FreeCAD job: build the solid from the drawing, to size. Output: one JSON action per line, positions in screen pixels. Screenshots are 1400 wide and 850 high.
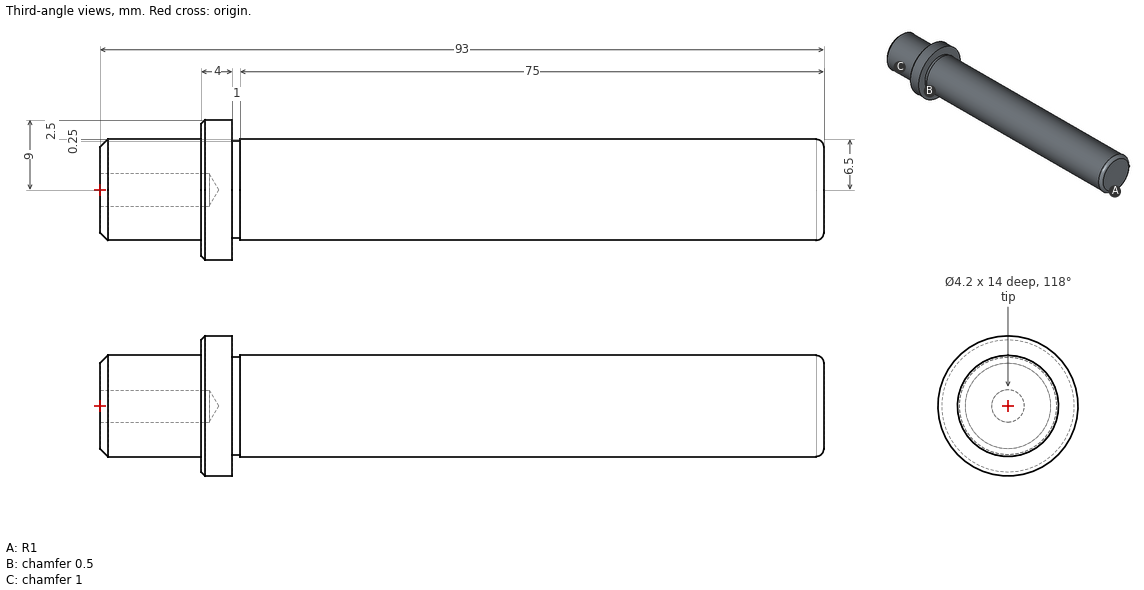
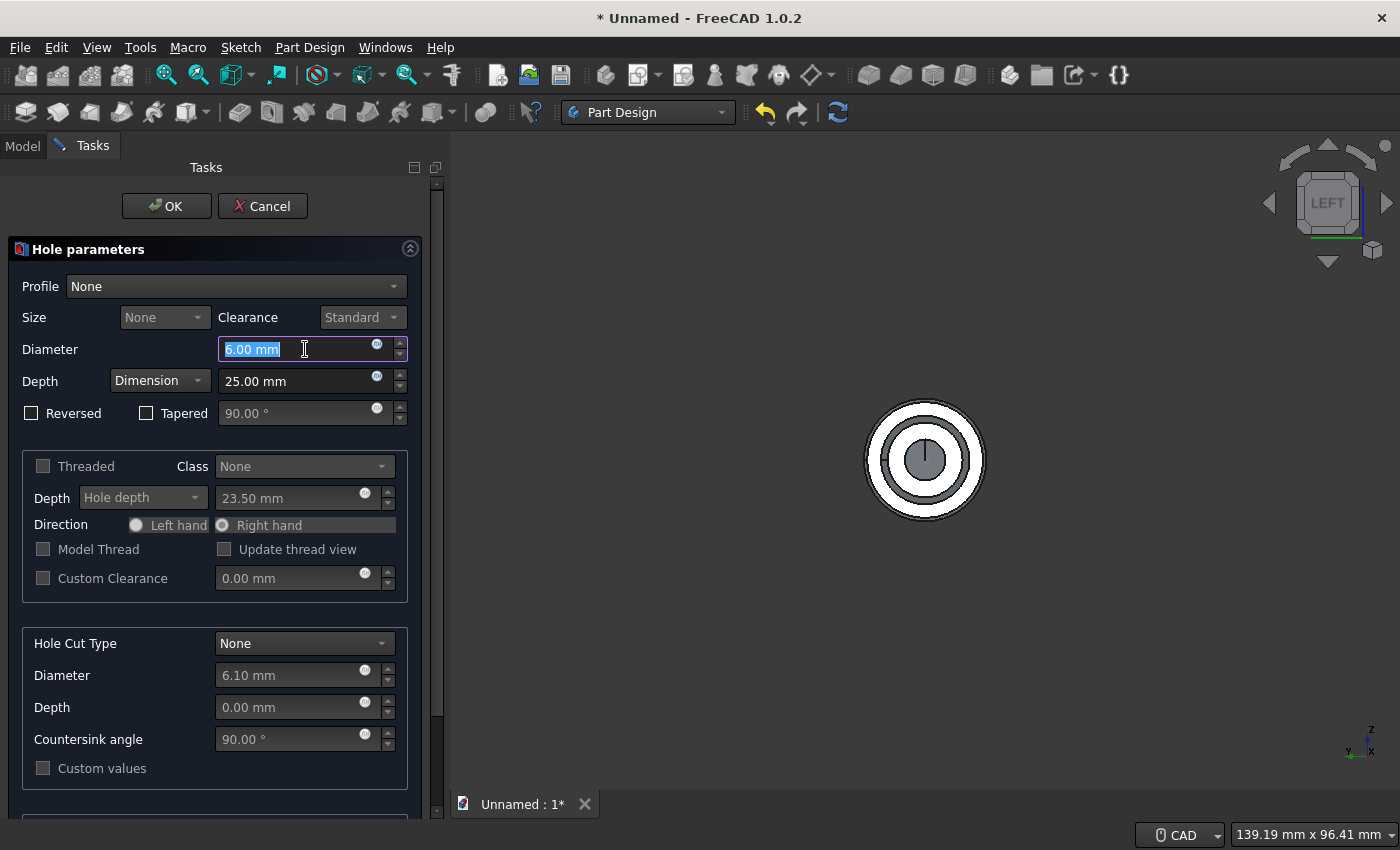
{"action": "type", "text": "4.2"}
{"action": "key", "text": "Tab"}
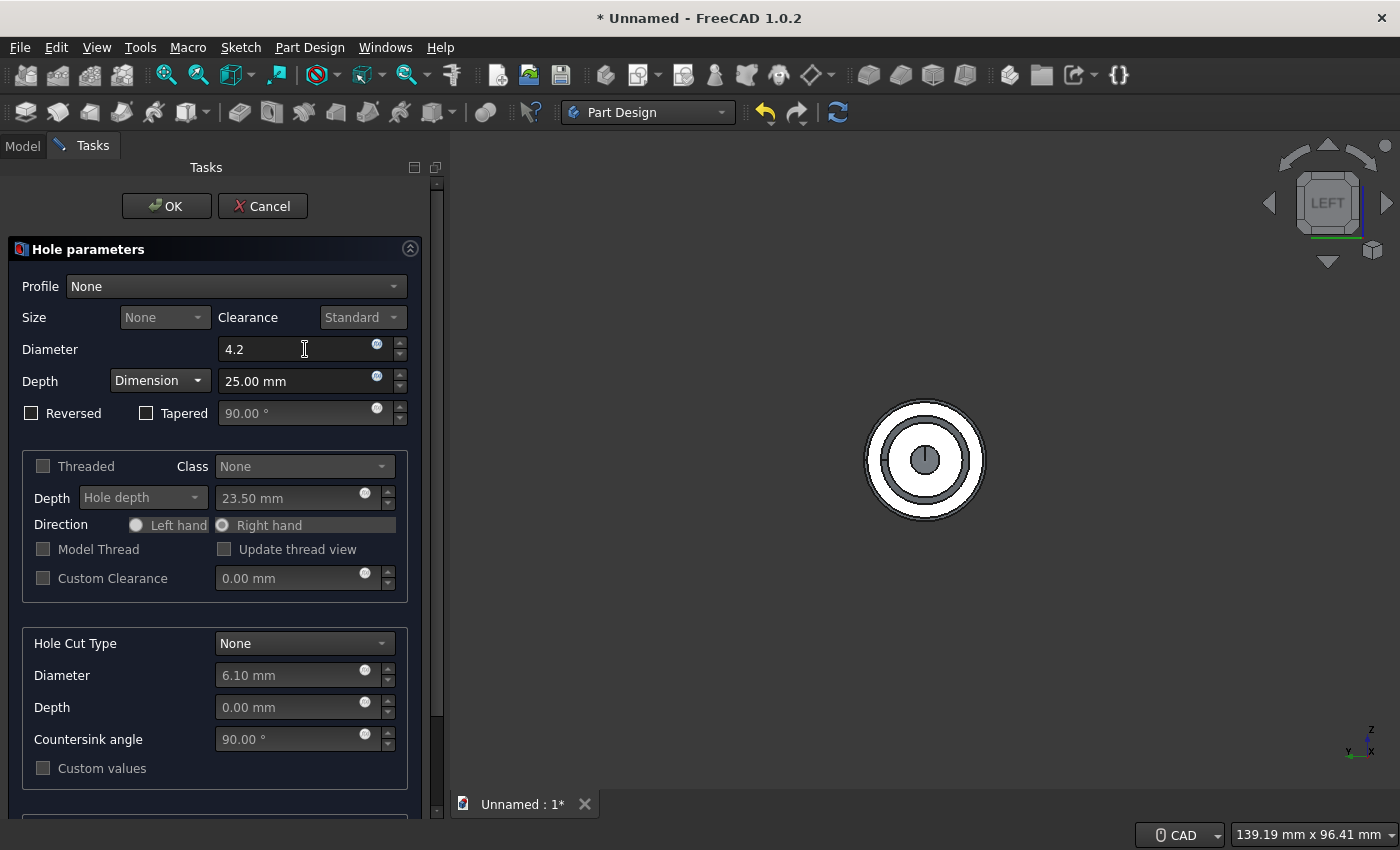
{"action": "triple_click", "coordinate": [305, 381]}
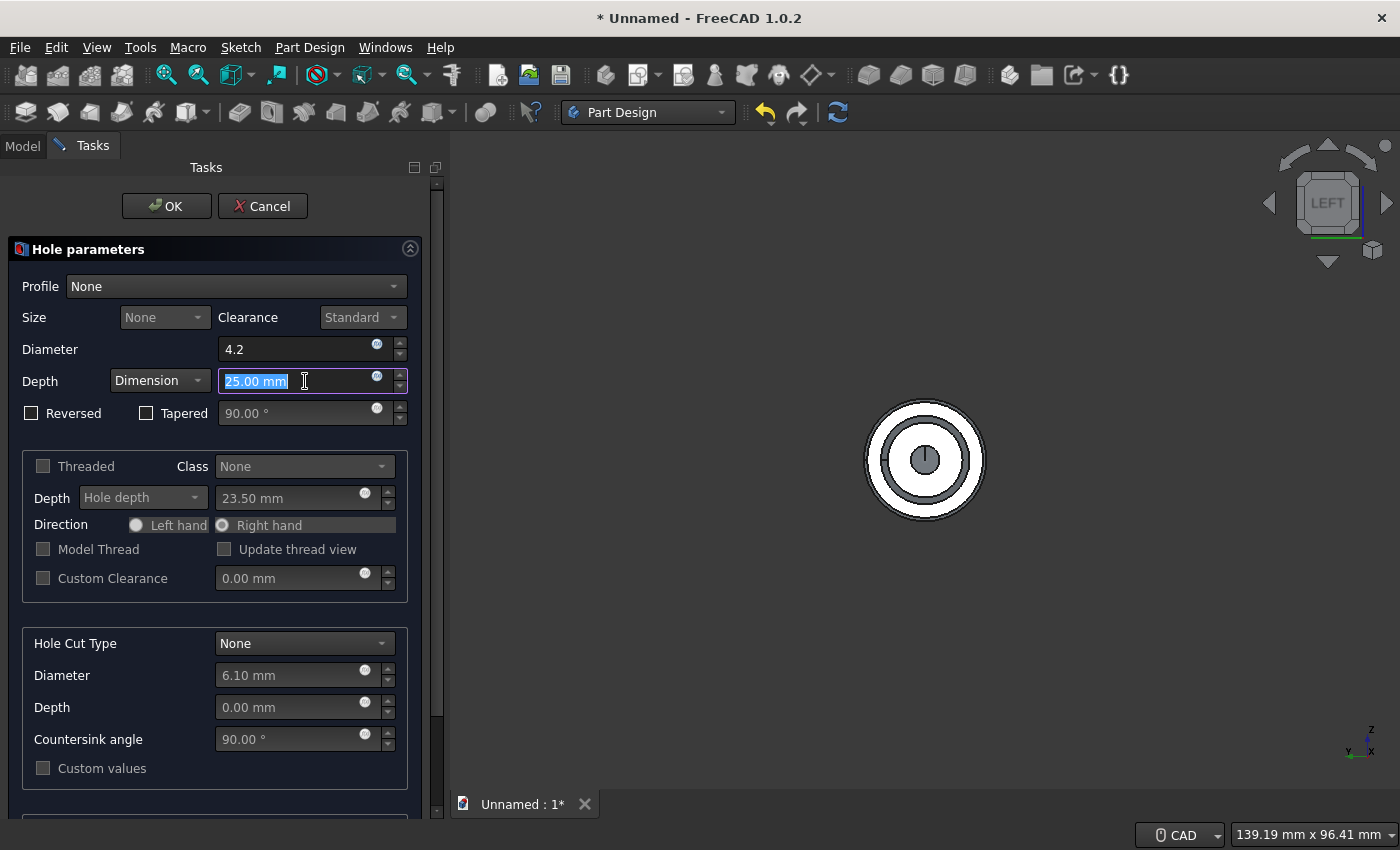
{"action": "type", "text": "14"}
{"action": "key", "text": "Tab"}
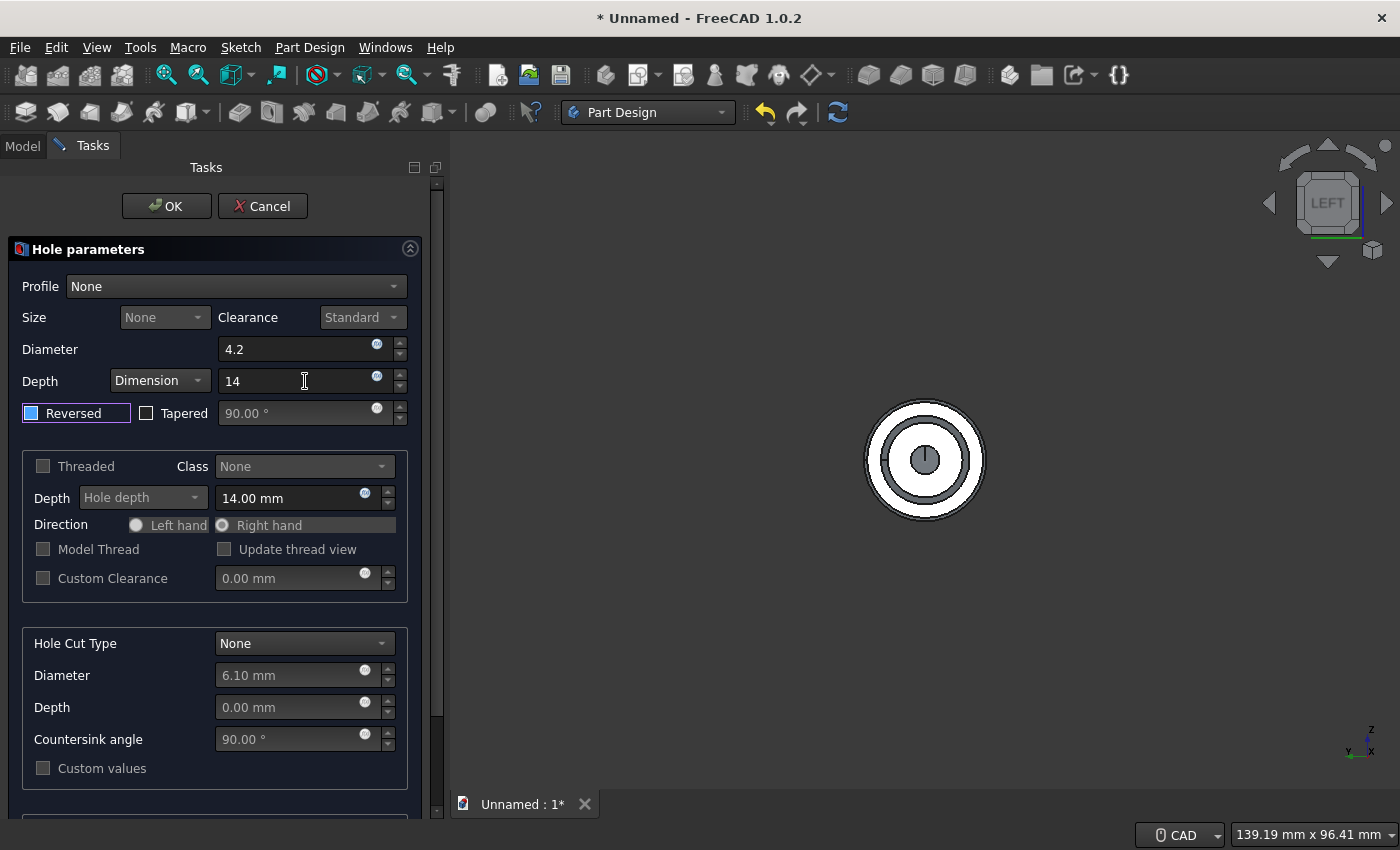
{"action": "left_click", "coordinate": [167, 206]}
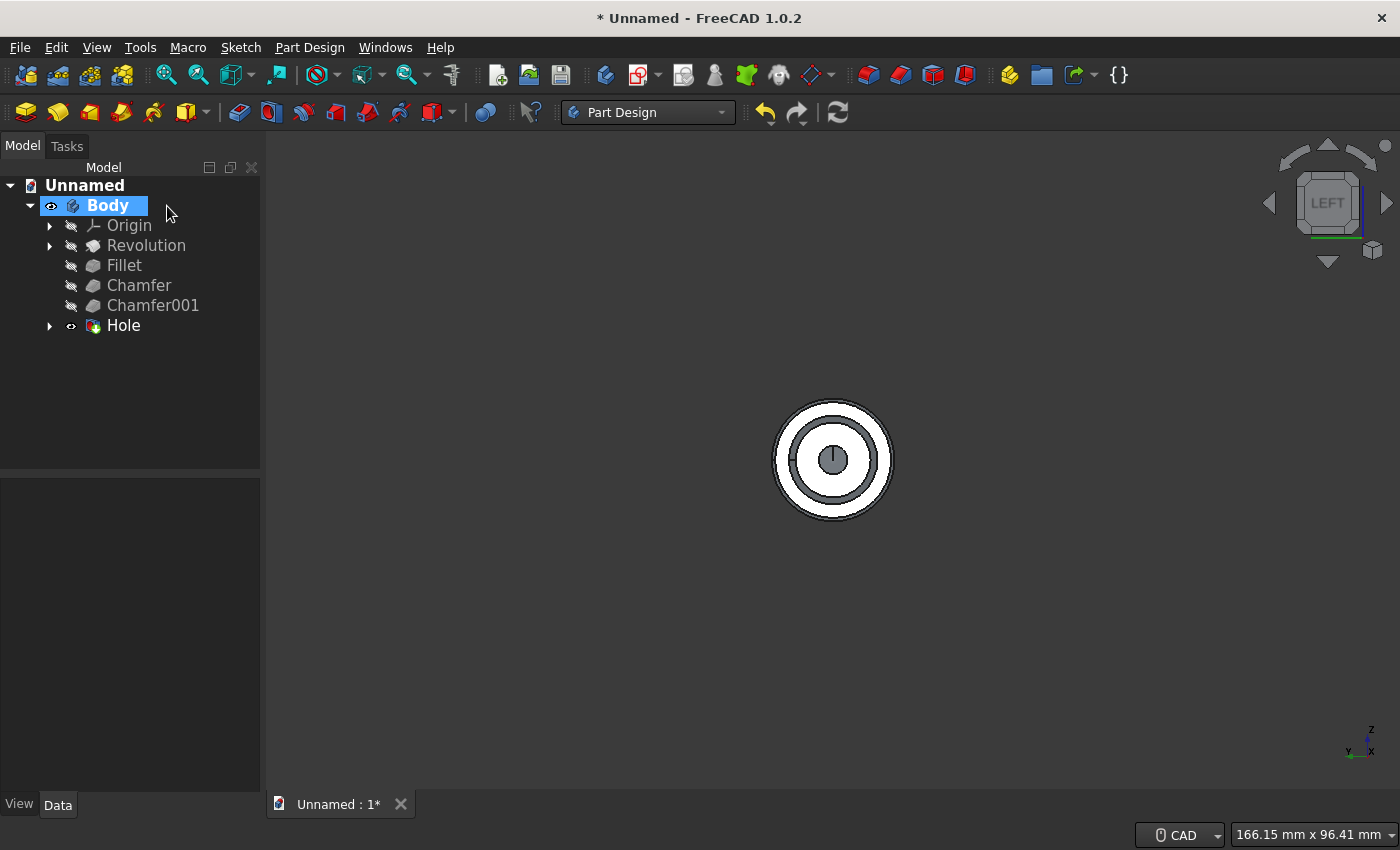
{"action": "key", "text": "0"}